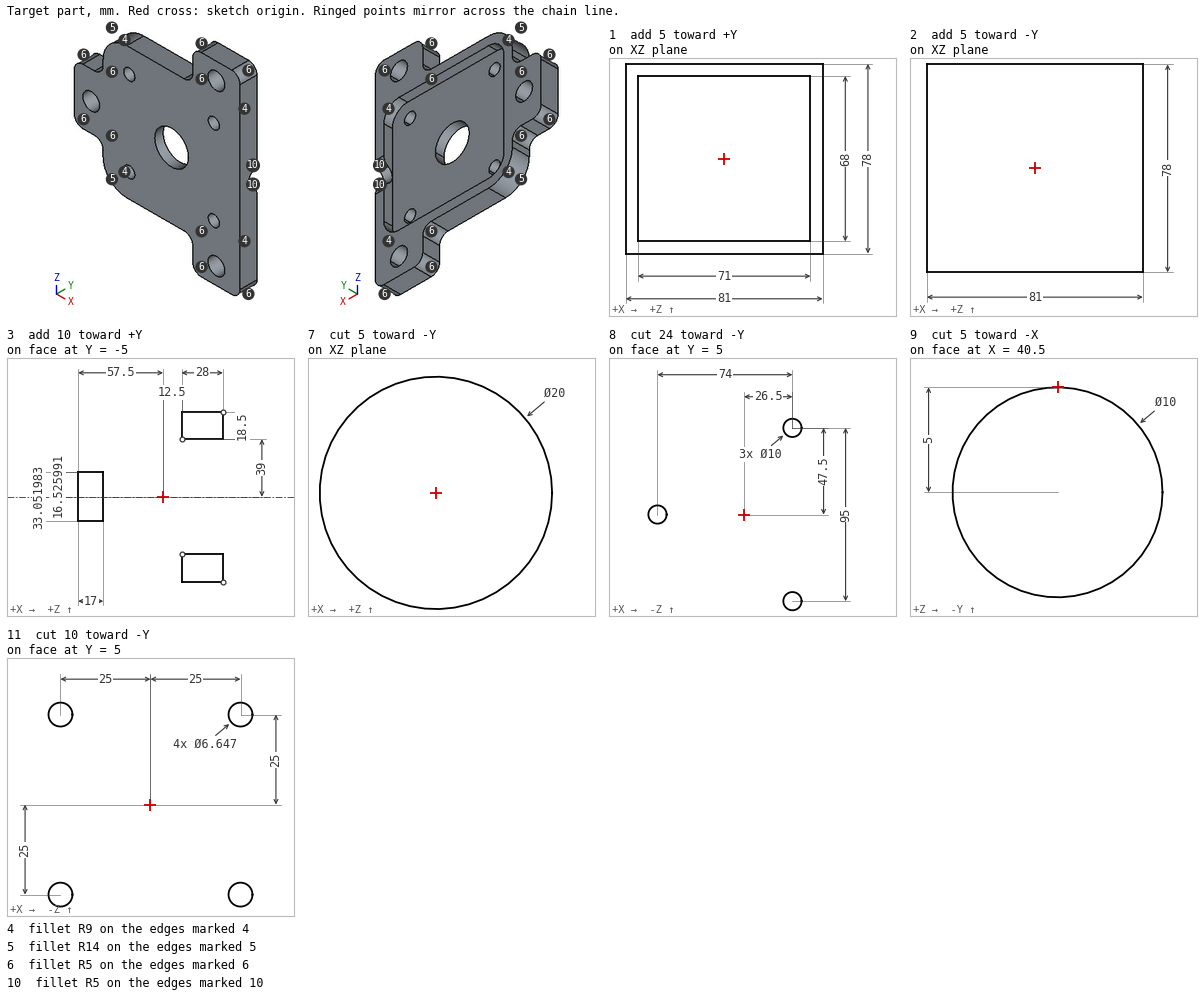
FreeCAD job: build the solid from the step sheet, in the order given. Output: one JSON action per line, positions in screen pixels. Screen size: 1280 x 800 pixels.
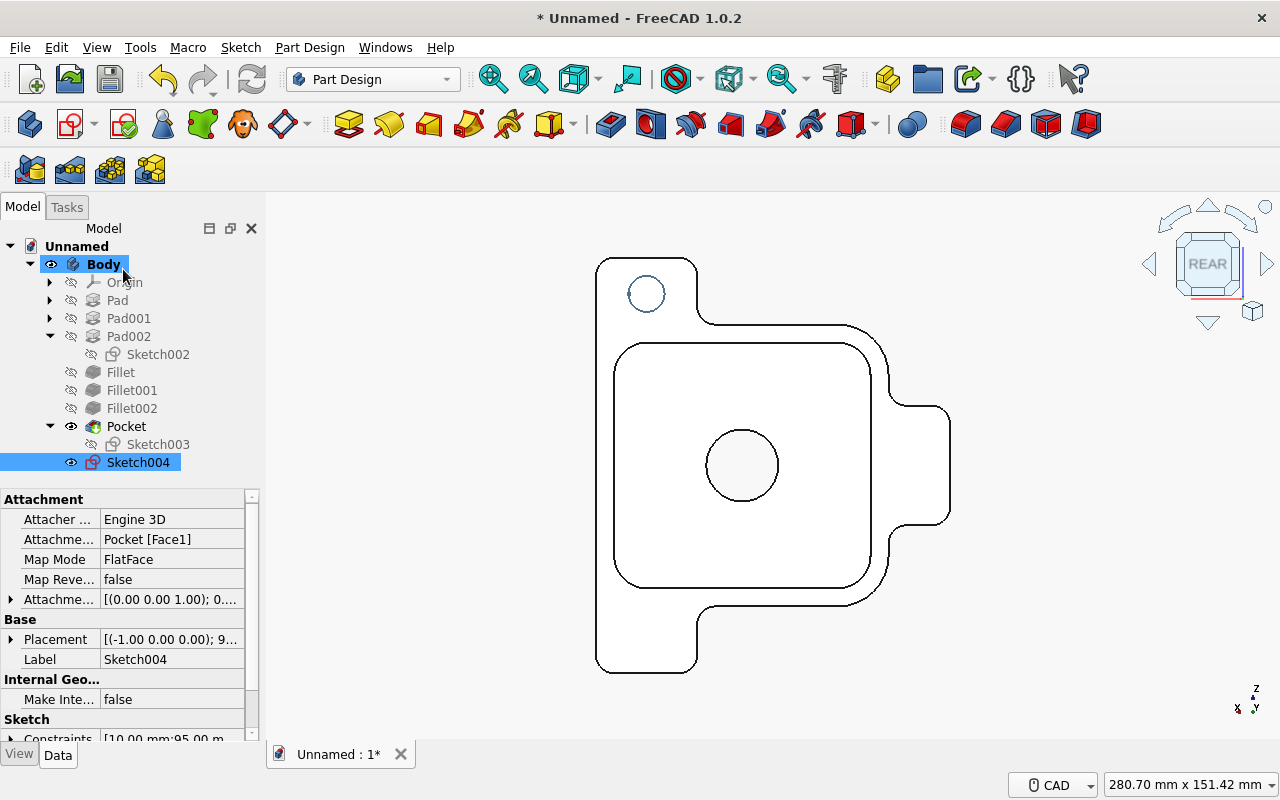
{"action": "left_click", "coordinate": [612, 124]}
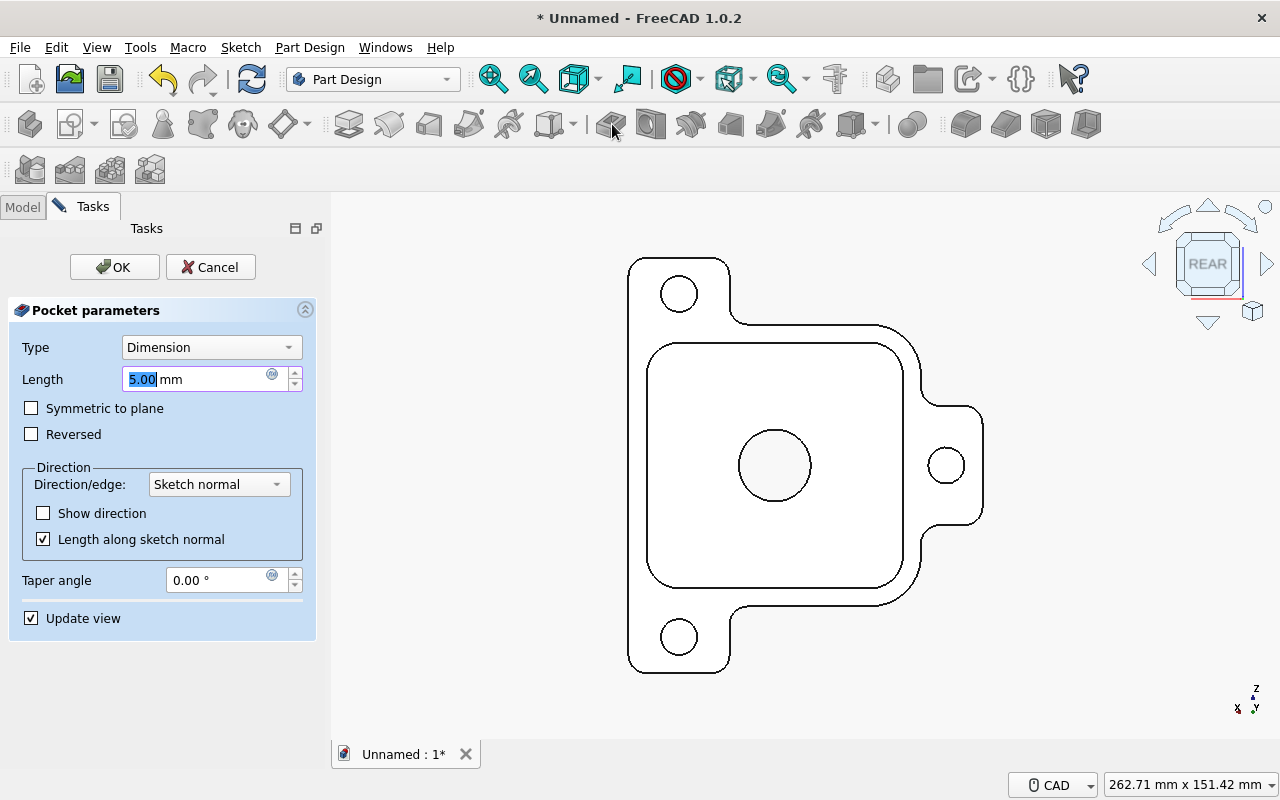
{"action": "type", "text": "24"}
{"action": "key", "text": "Tab"}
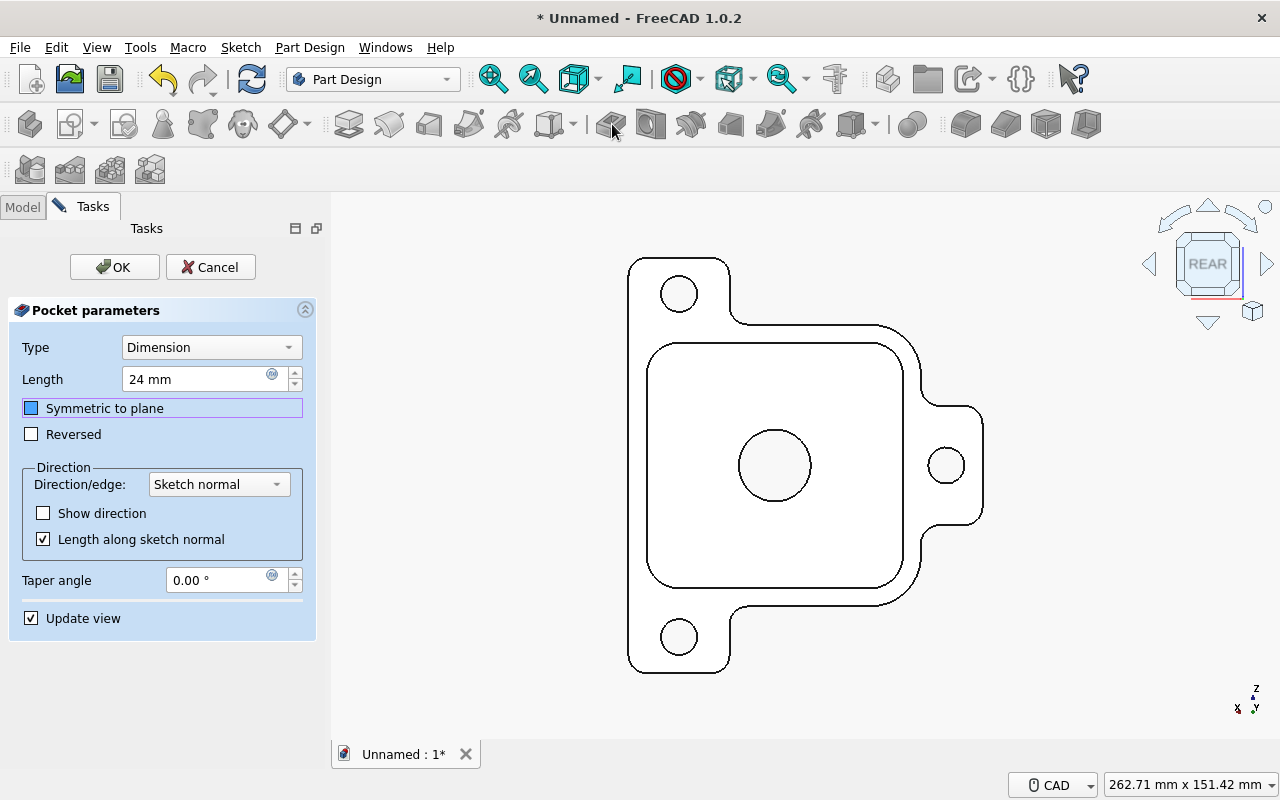
{"action": "left_click", "coordinate": [115, 267]}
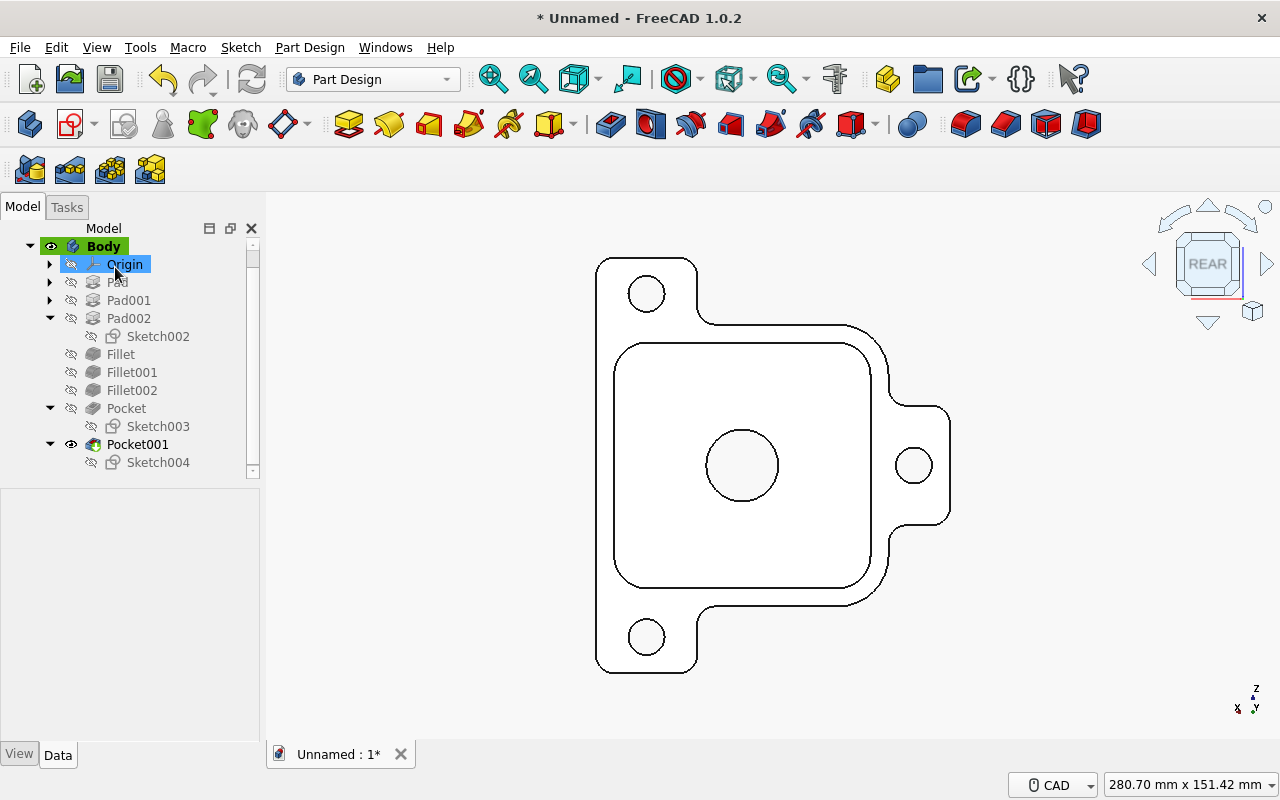
{"action": "key", "text": "0"}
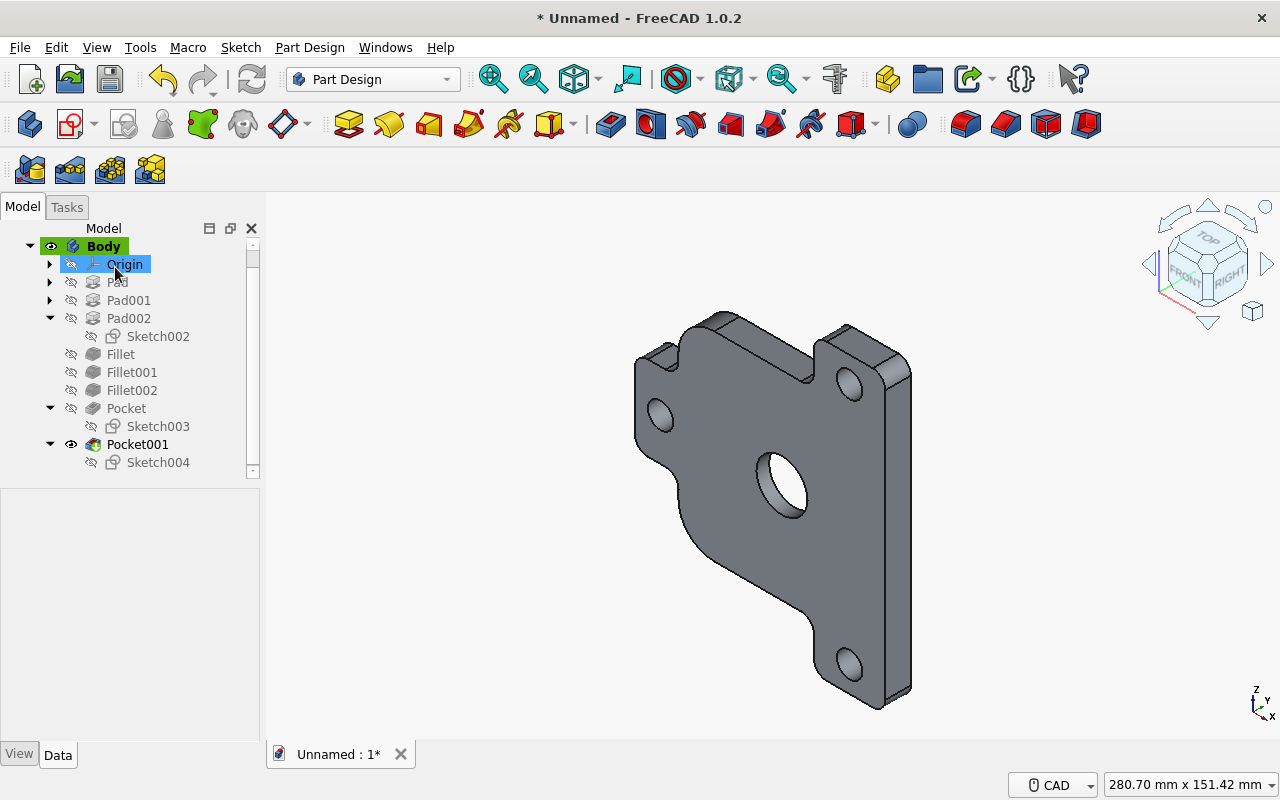
{"action": "left_click", "coordinate": [898, 537]}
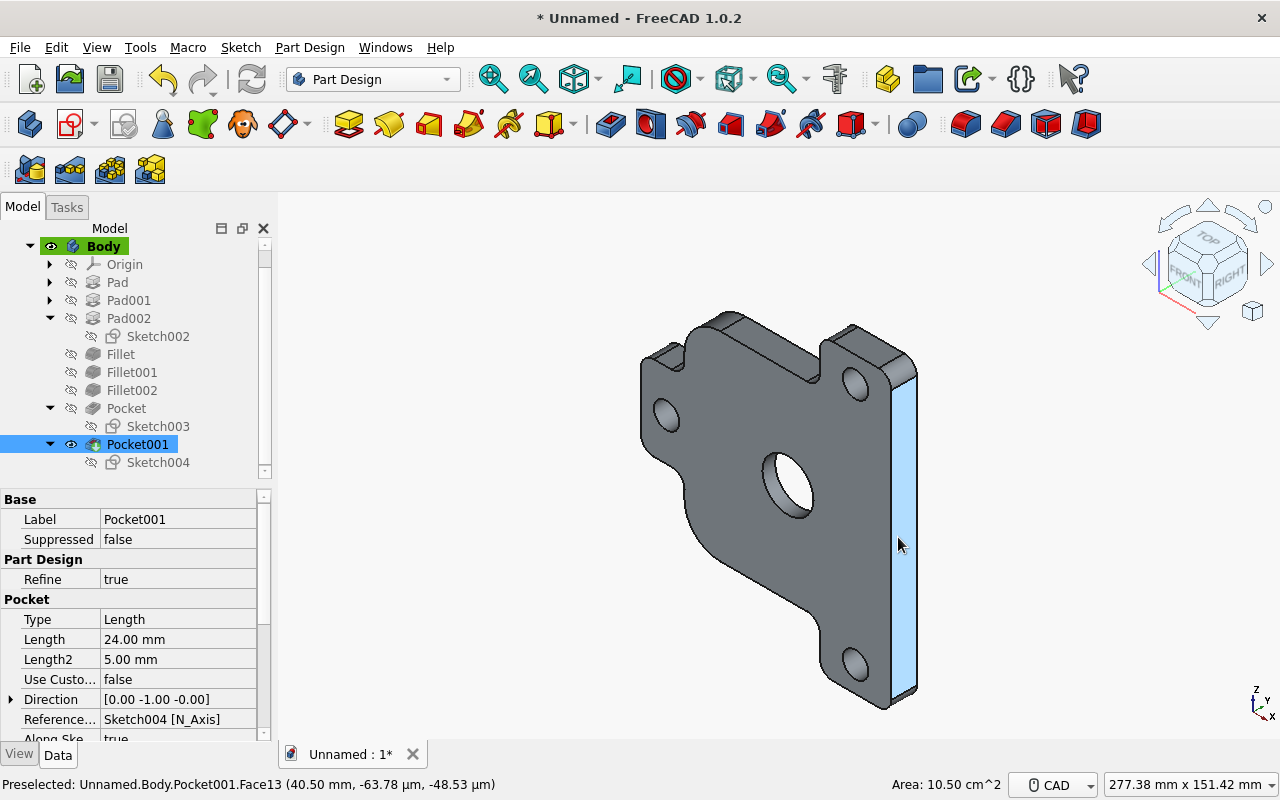
{"action": "left_click", "coordinate": [70, 124]}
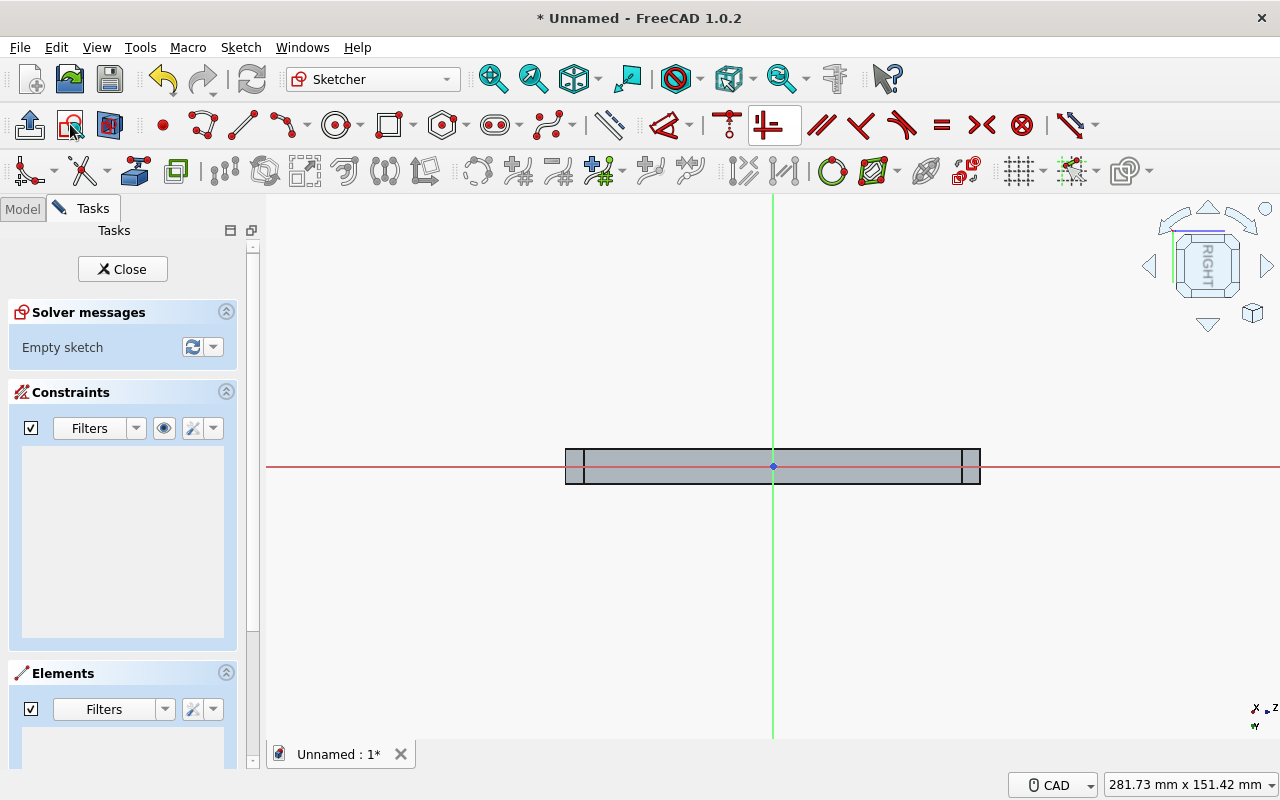
{"action": "scroll", "coordinate": [782, 487], "scroll_direction": "up", "scroll_amount": 11}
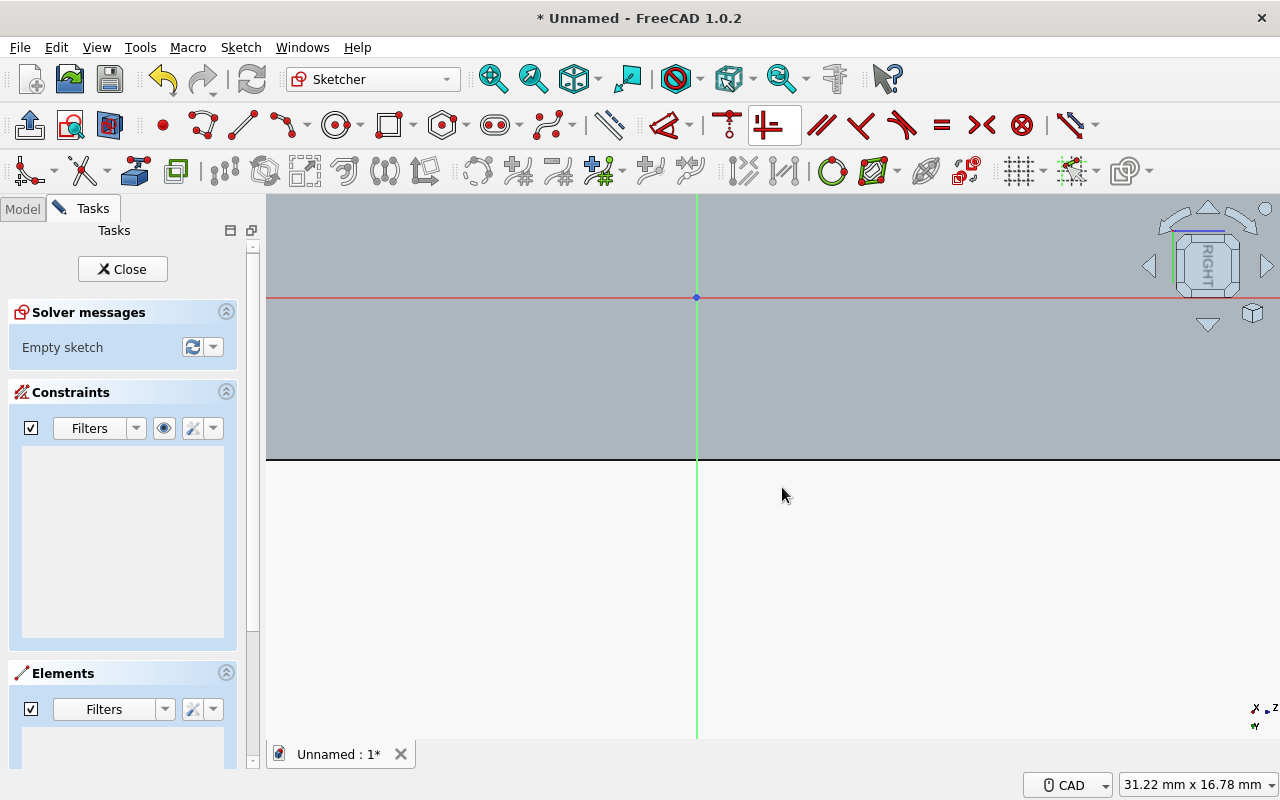
{"action": "key", "text": "g c"}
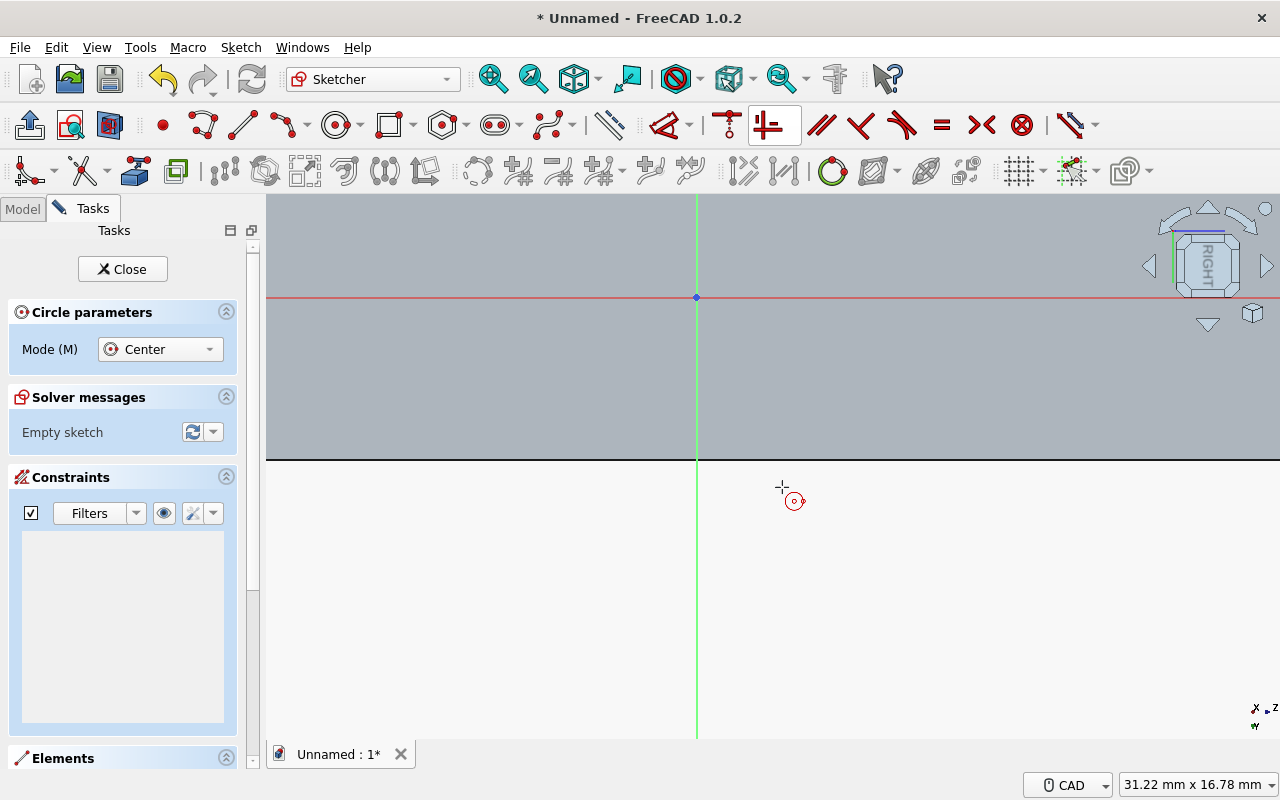
{"action": "left_click", "coordinate": [697, 460]}
{"action": "left_click", "coordinate": [812, 345]}
{"action": "key", "text": "Escape"}